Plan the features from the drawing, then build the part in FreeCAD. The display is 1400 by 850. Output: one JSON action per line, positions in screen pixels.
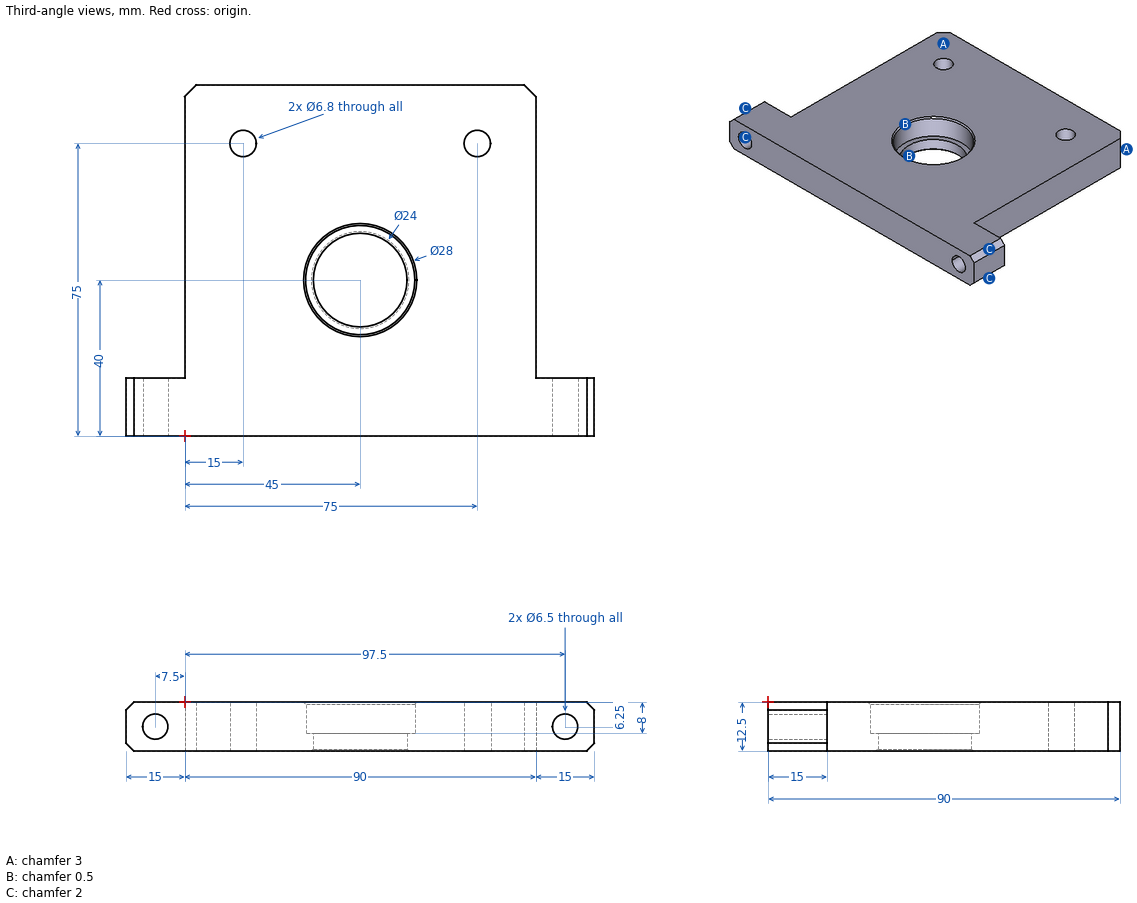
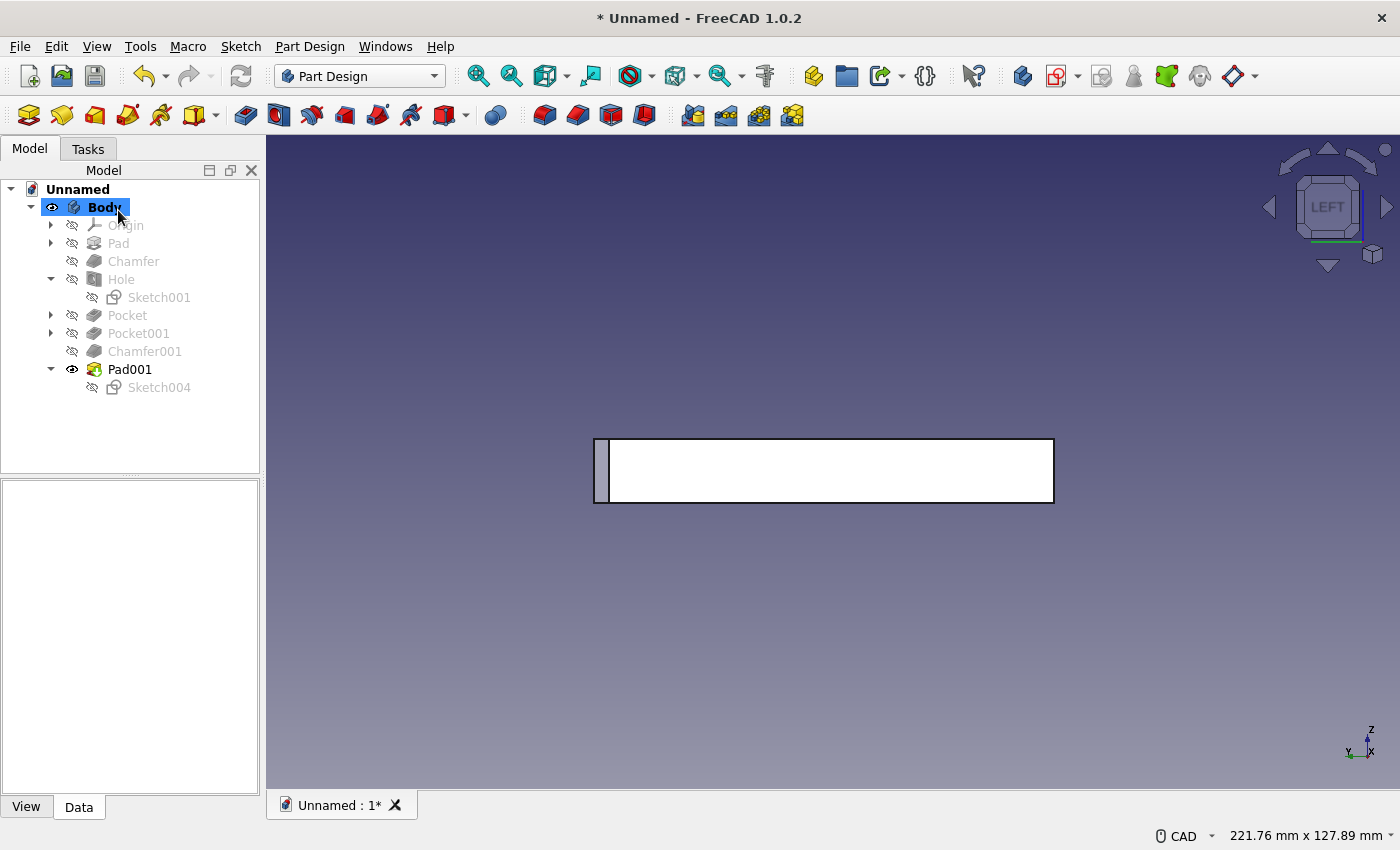
{"action": "left_click", "coordinate": [479, 76]}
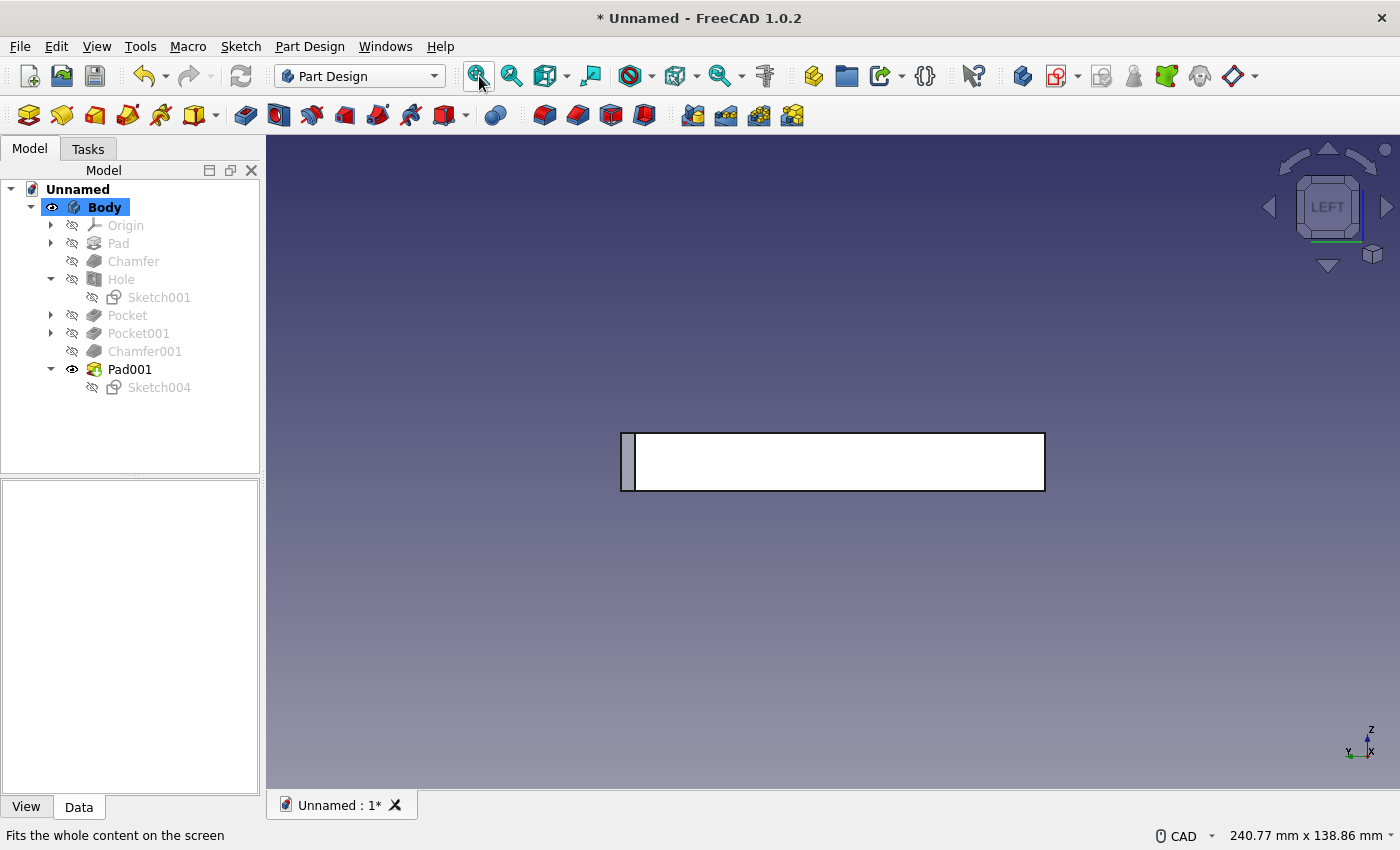
{"action": "left_click", "coordinate": [723, 461]}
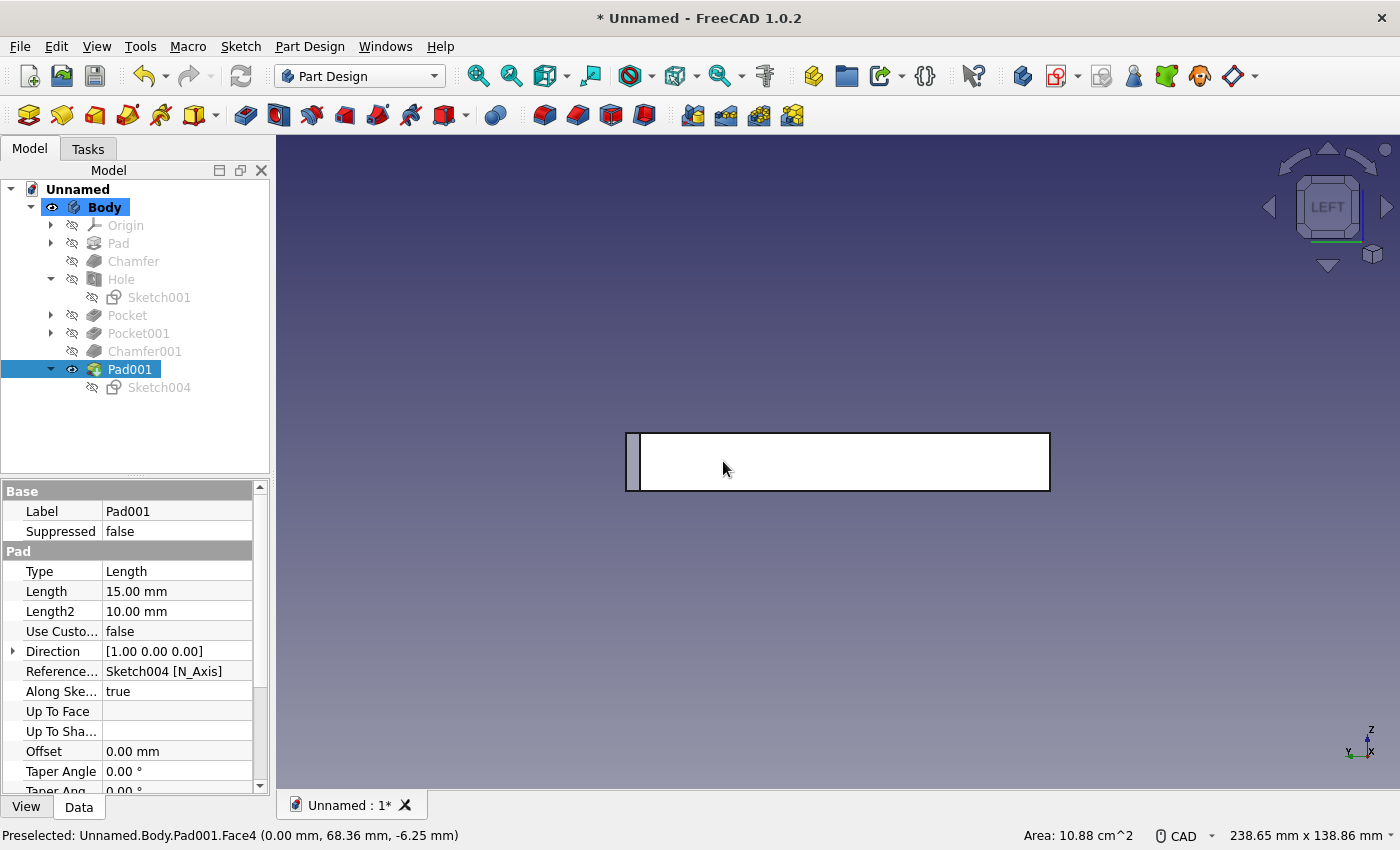
{"action": "left_click", "coordinate": [1056, 76]}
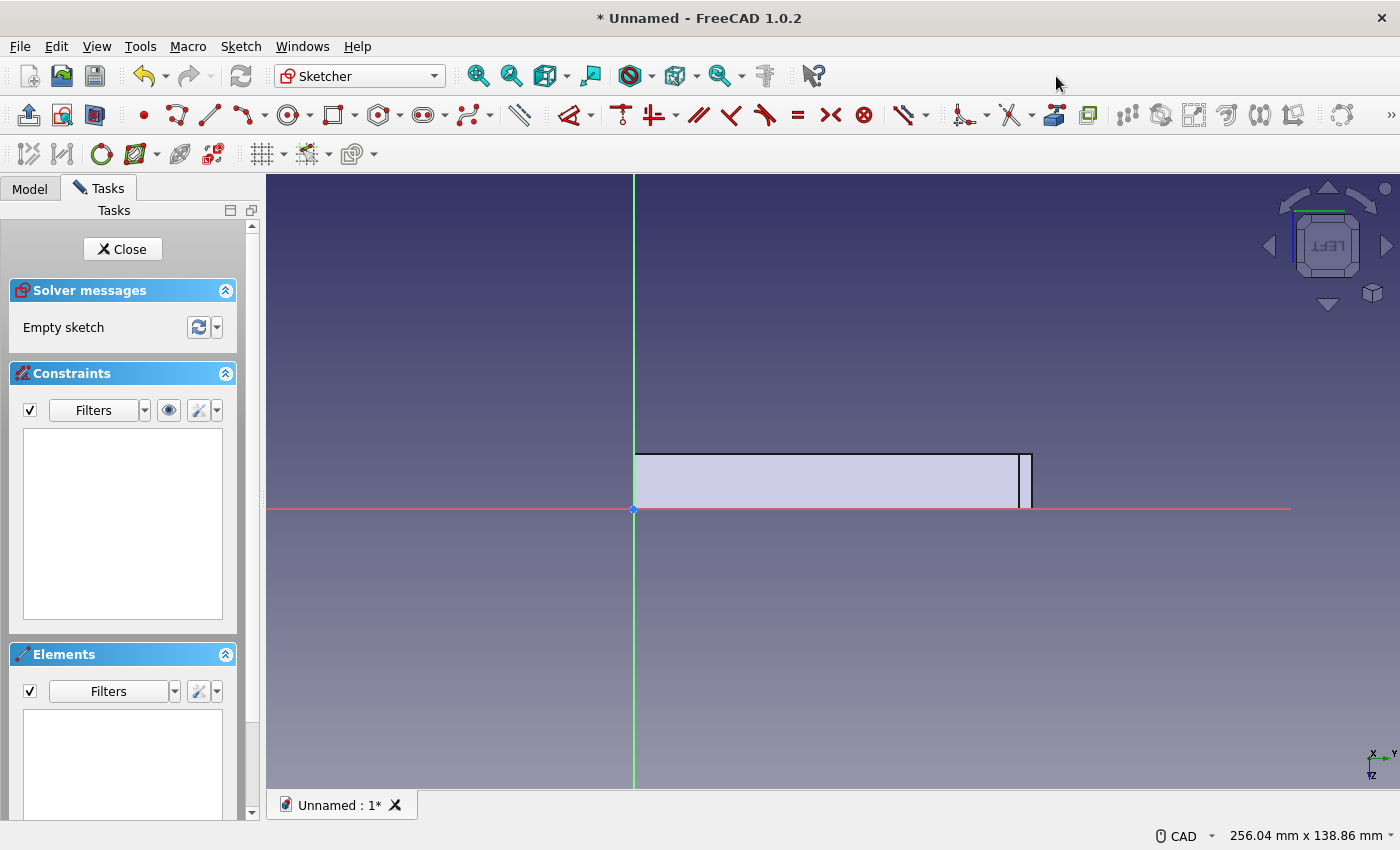
{"action": "scroll", "coordinate": [652, 482], "scroll_direction": "up", "scroll_amount": 10}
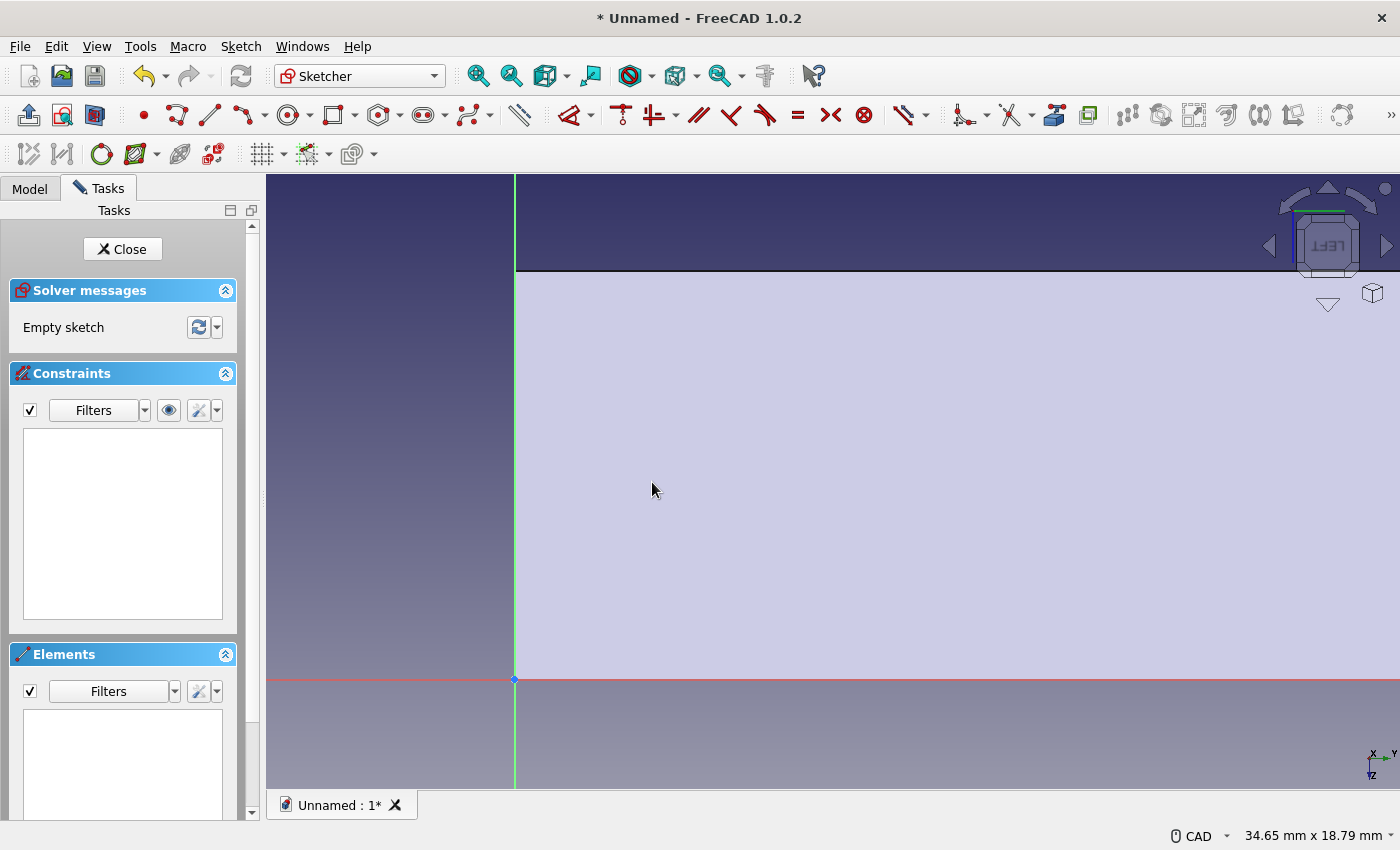
{"action": "left_click", "coordinate": [332, 116]}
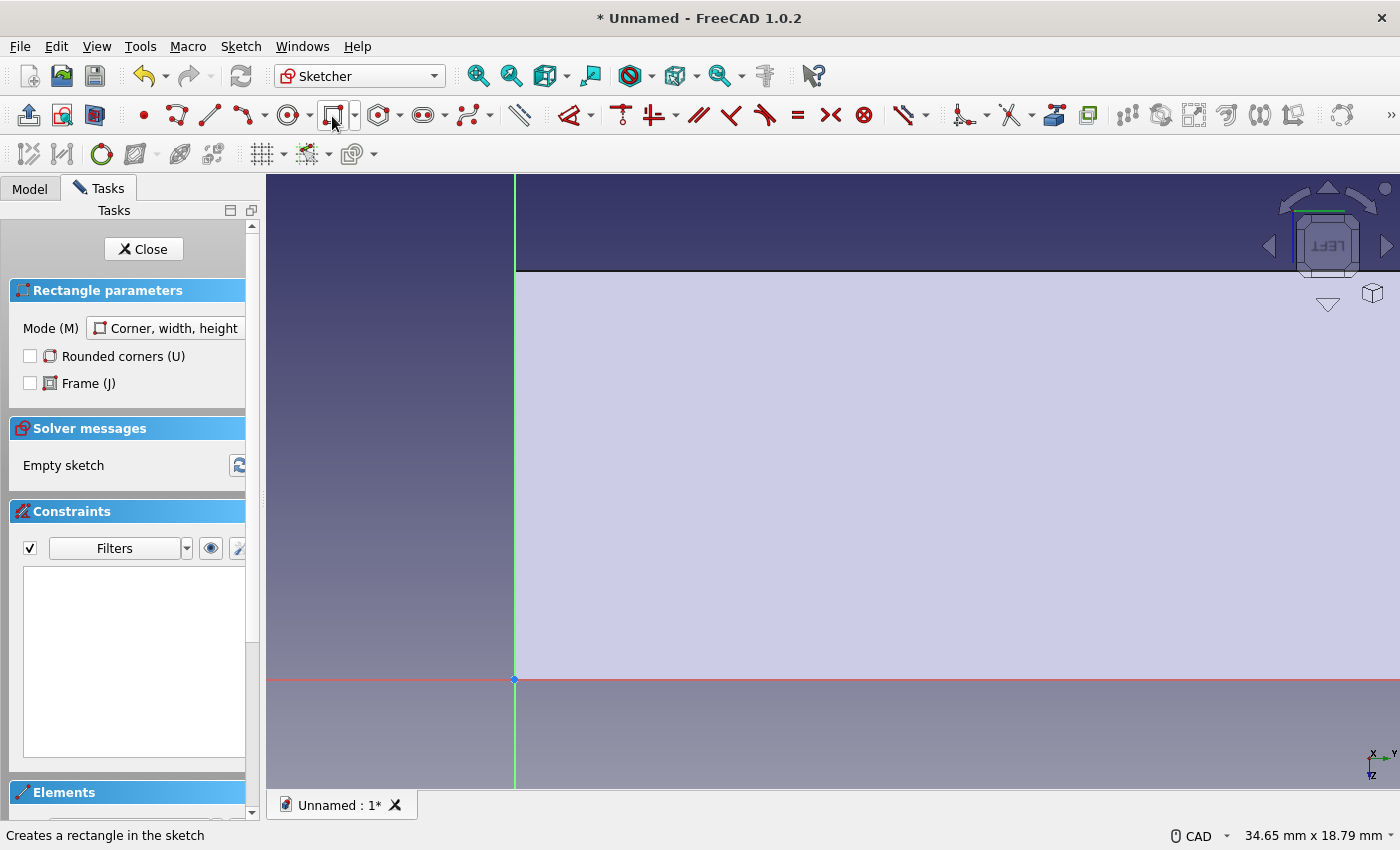
{"action": "left_click", "coordinate": [515, 680]}
{"action": "left_click", "coordinate": [1005, 271]}
{"action": "key", "text": "Escape"}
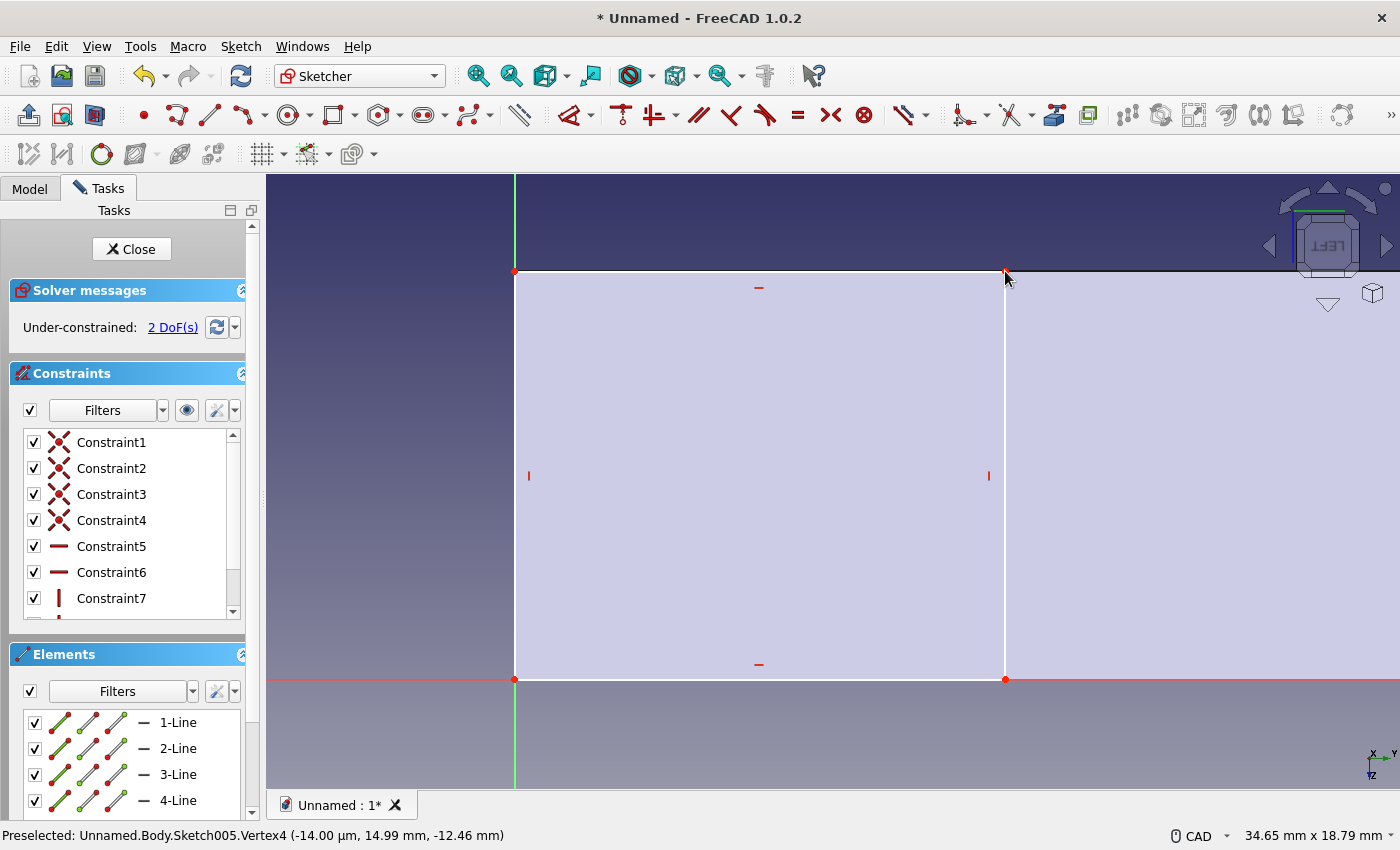
{"action": "left_click", "coordinate": [568, 116]}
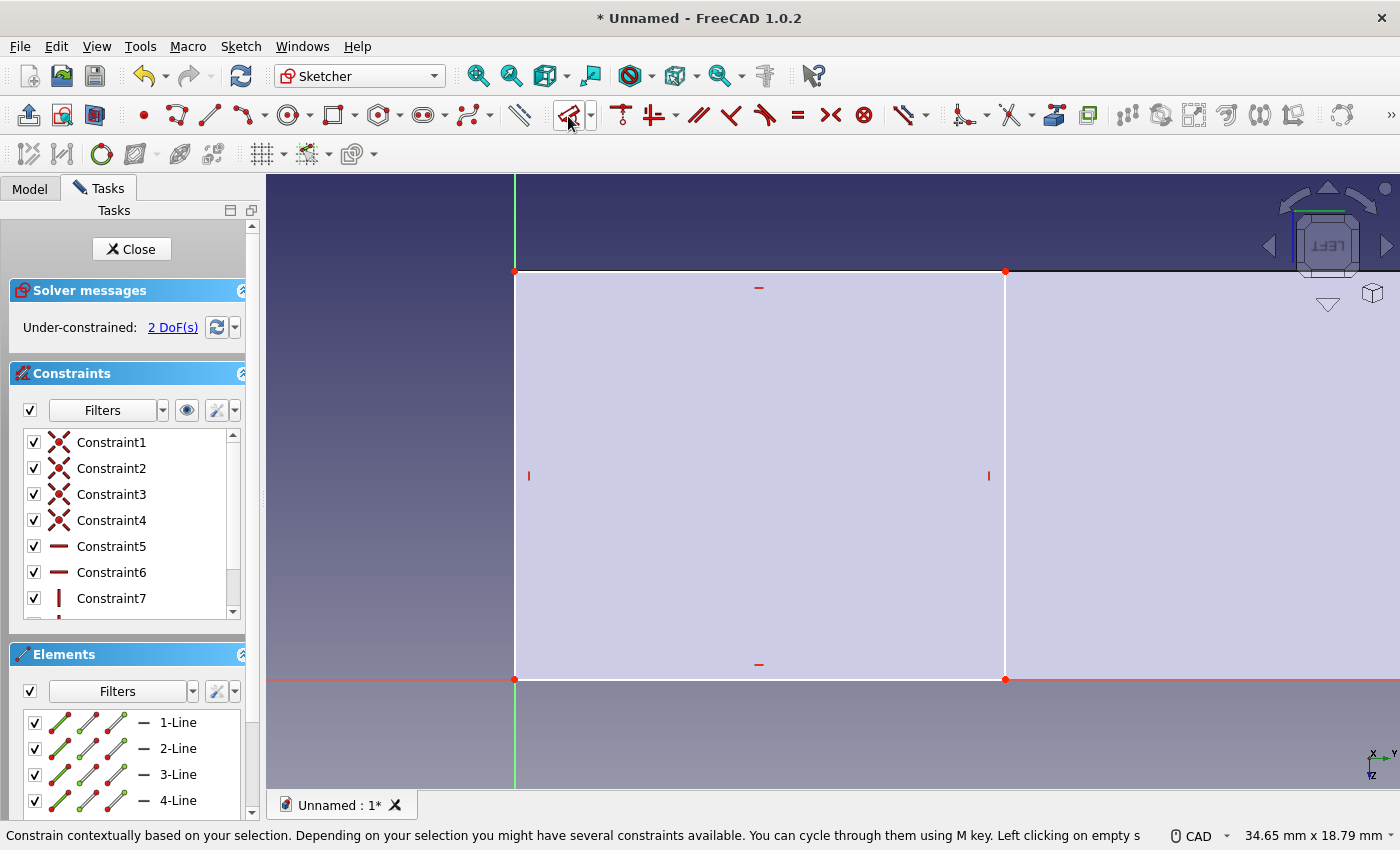
{"action": "left_click", "coordinate": [662, 680]}
{"action": "left_click", "coordinate": [760, 714]}